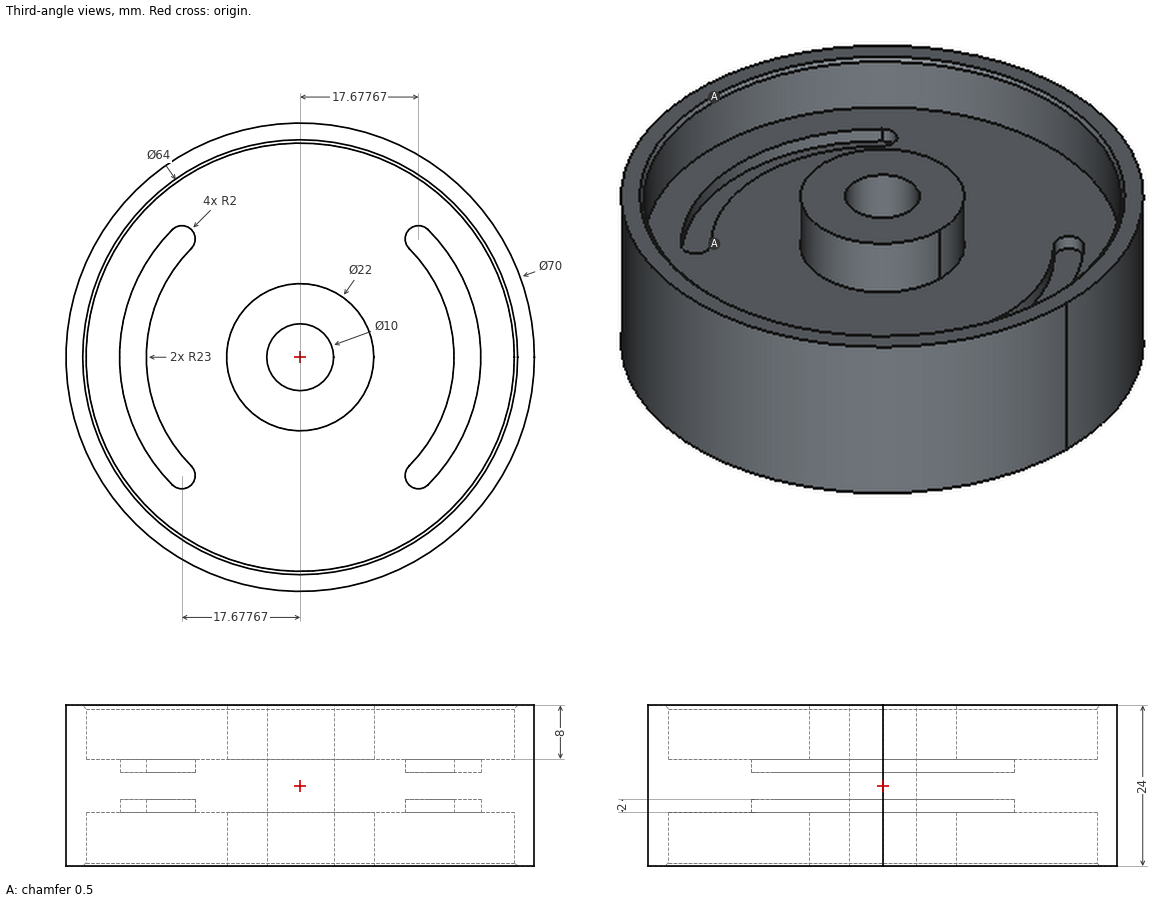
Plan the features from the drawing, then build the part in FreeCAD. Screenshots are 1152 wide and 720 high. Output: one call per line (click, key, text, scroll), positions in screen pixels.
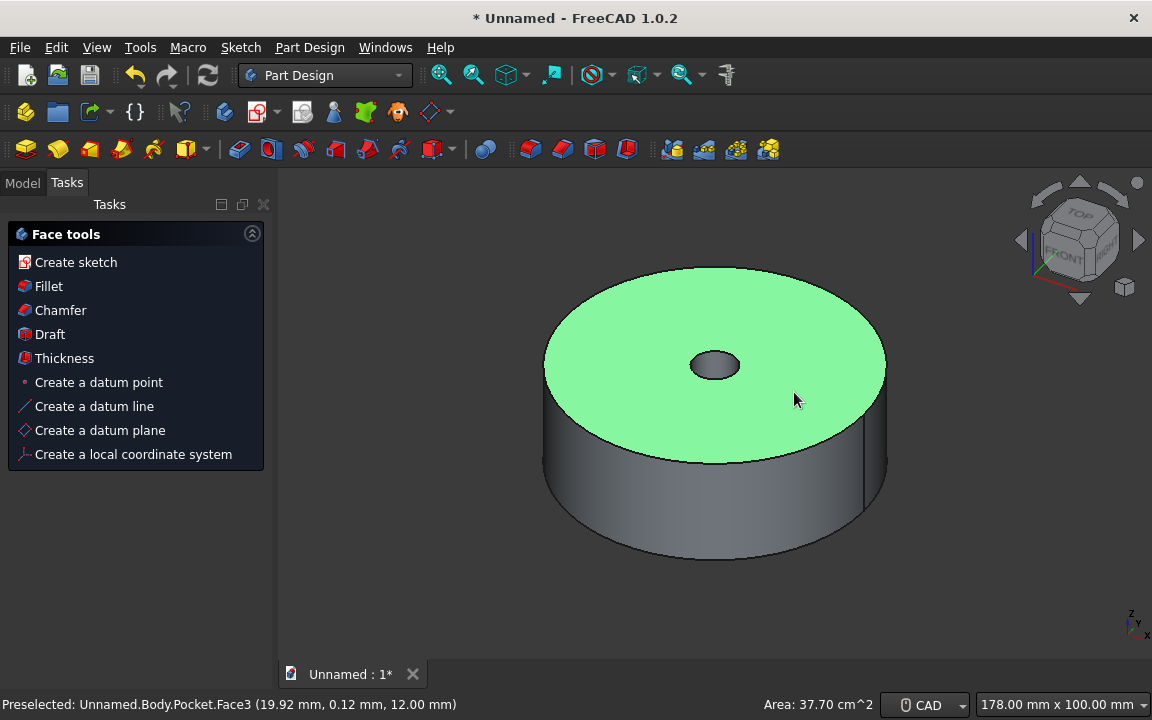
click(258, 112)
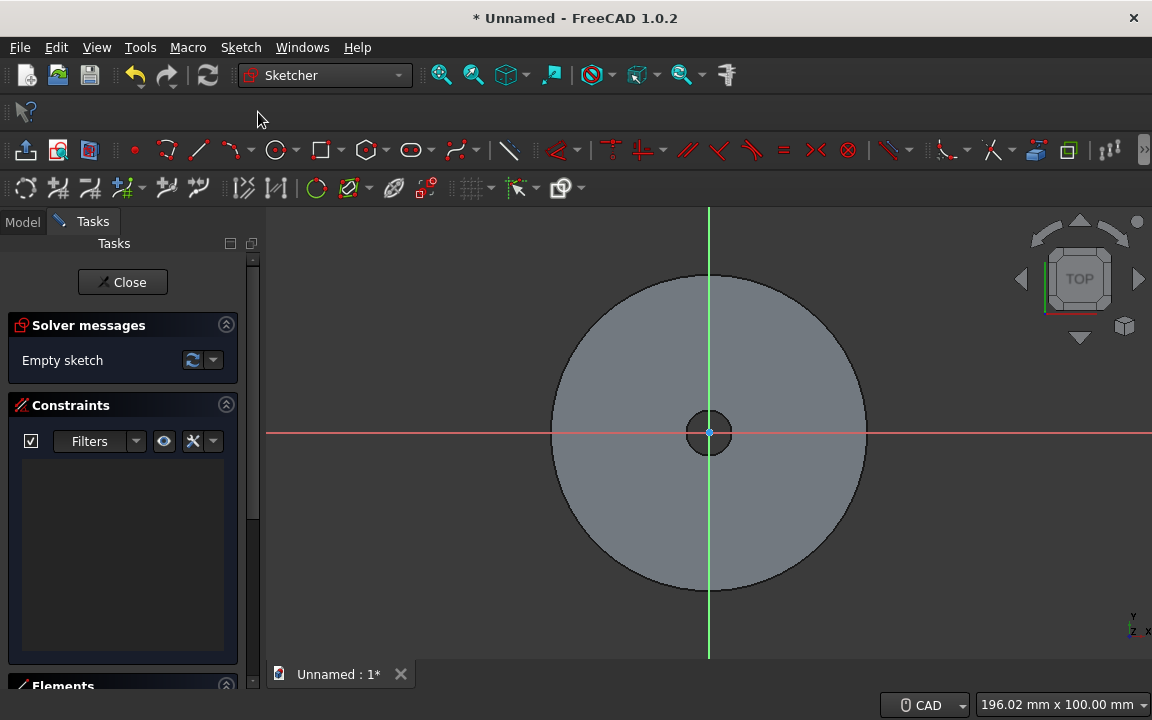
key(g)
key(c)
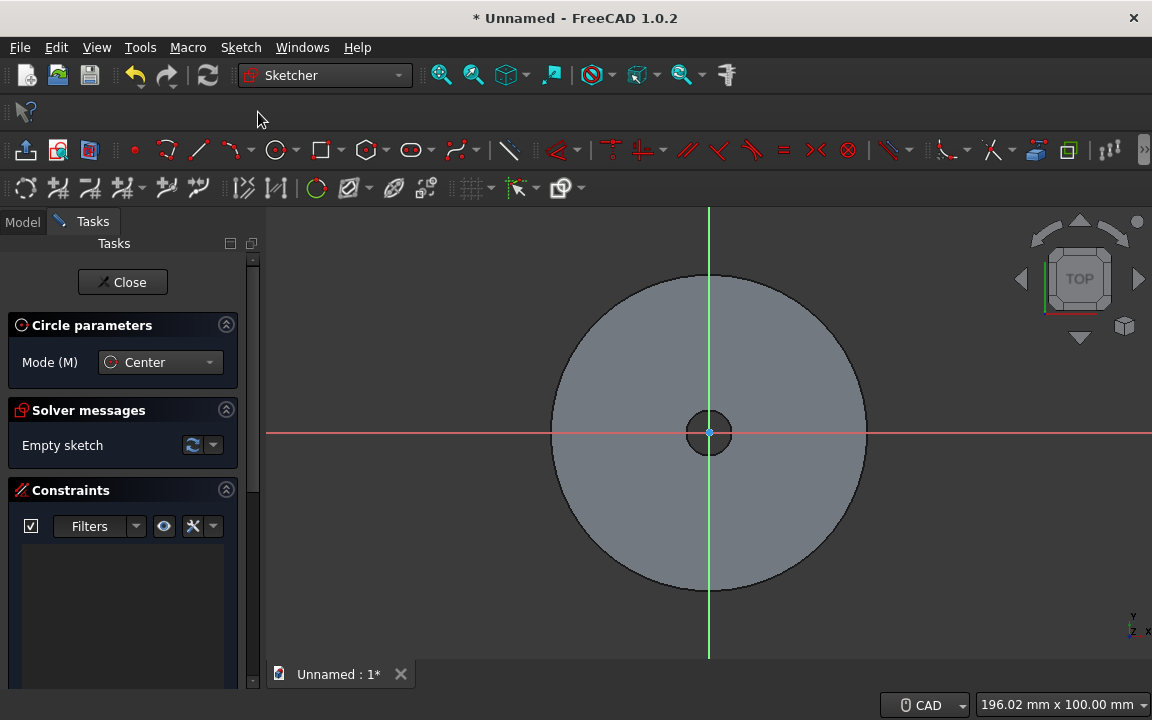
click(709, 433)
move(811, 331)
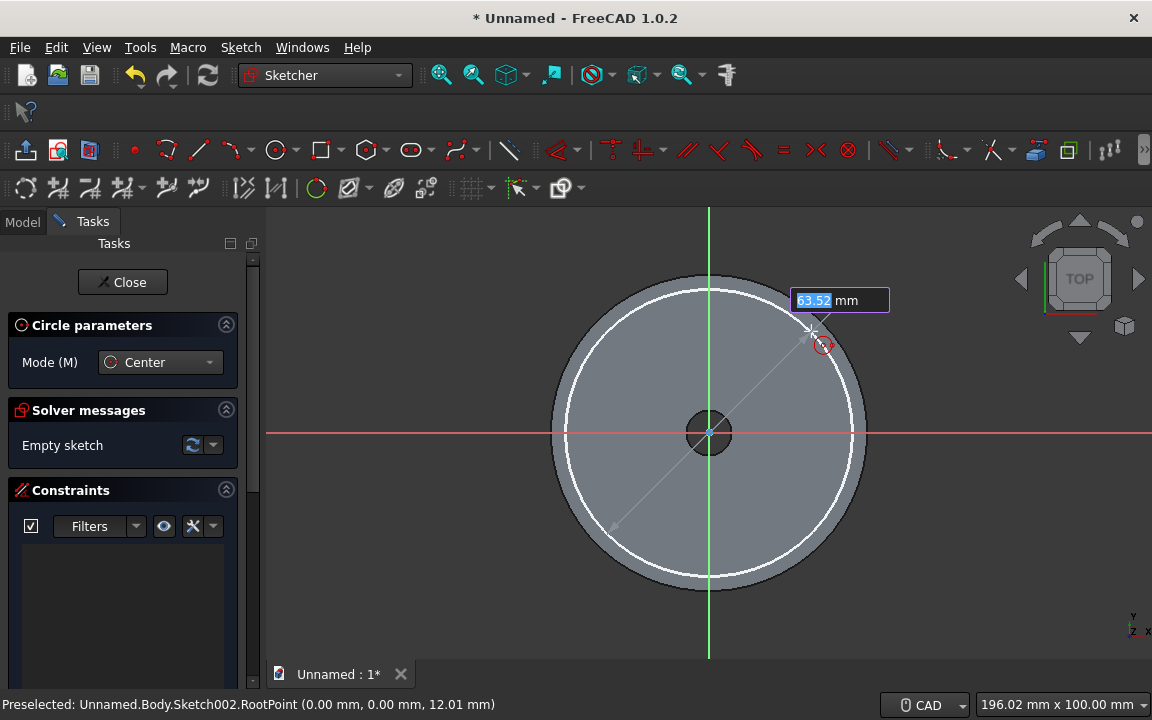
text(64)
key(Return)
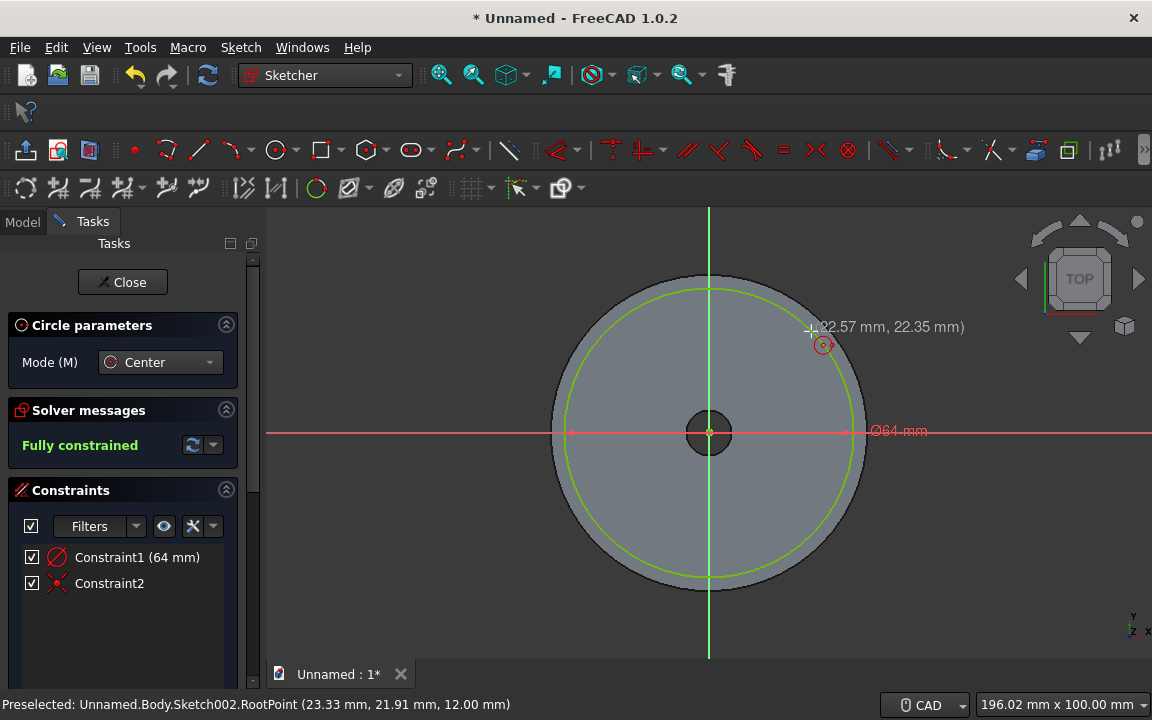
click(709, 433)
move(744, 398)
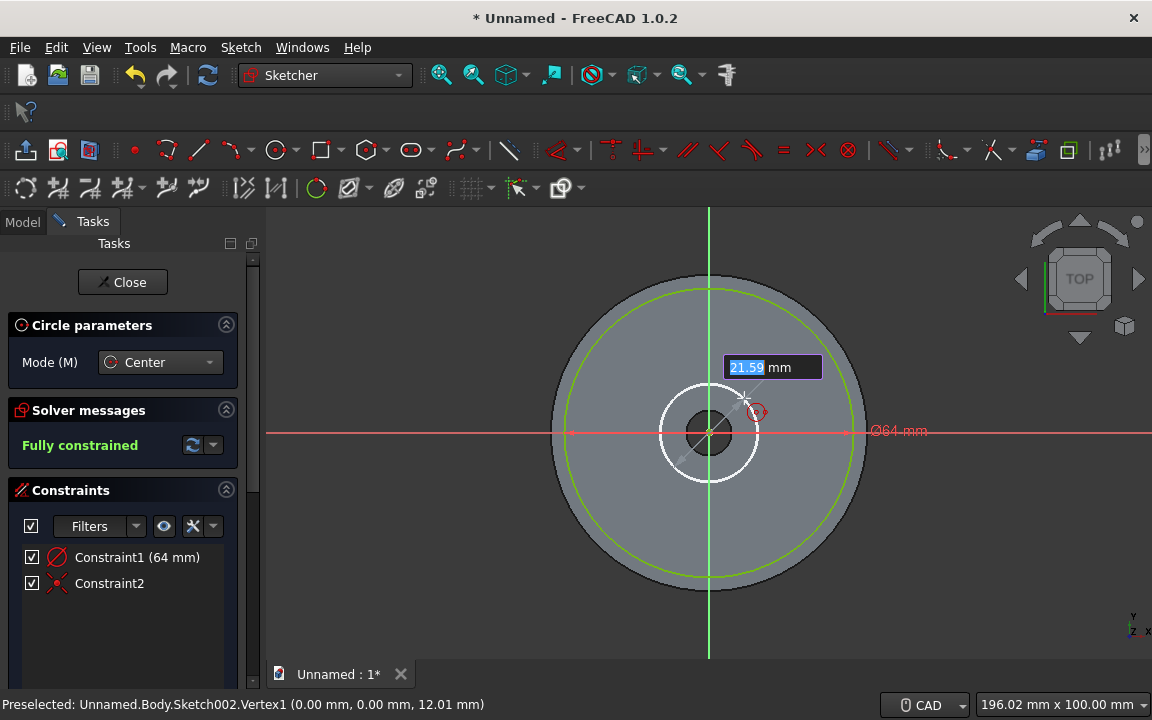
text(22)
key(Return)
key(Escape)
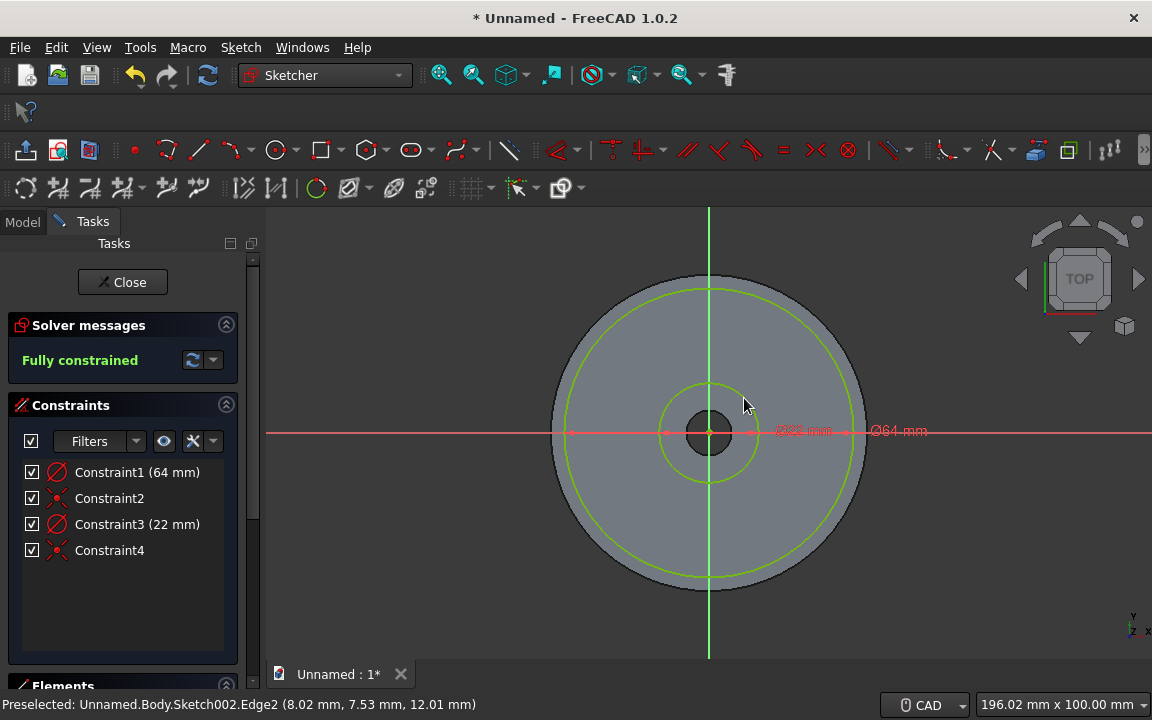
click(123, 282)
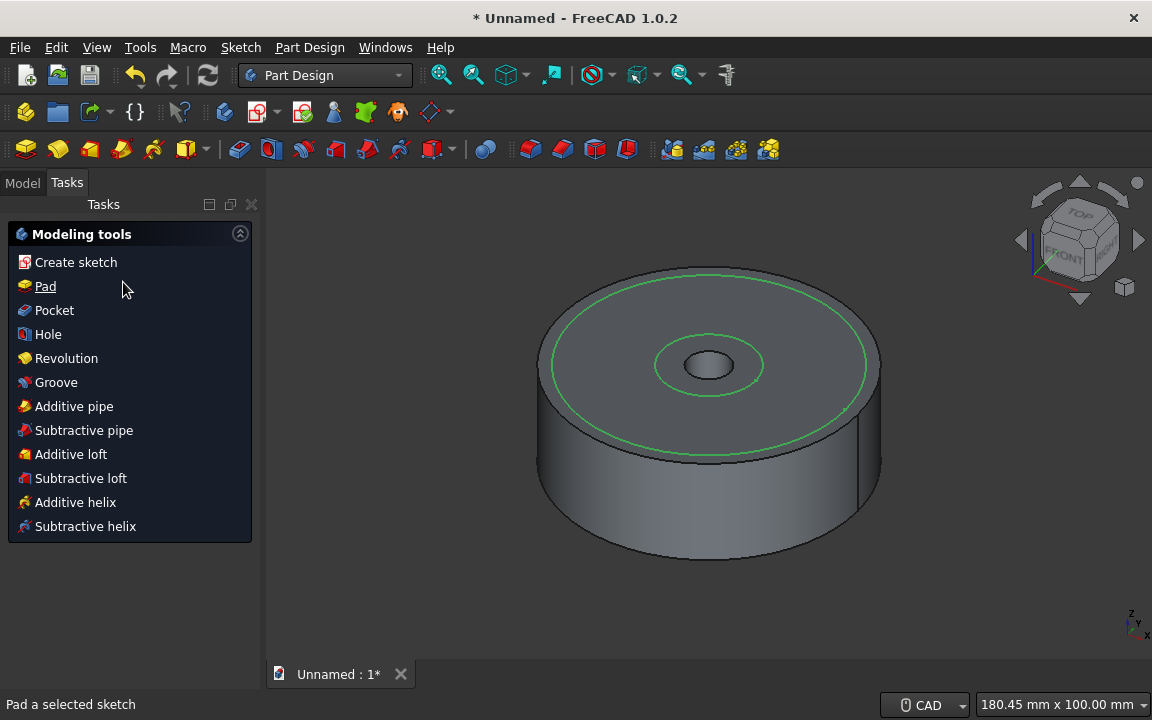
click(240, 150)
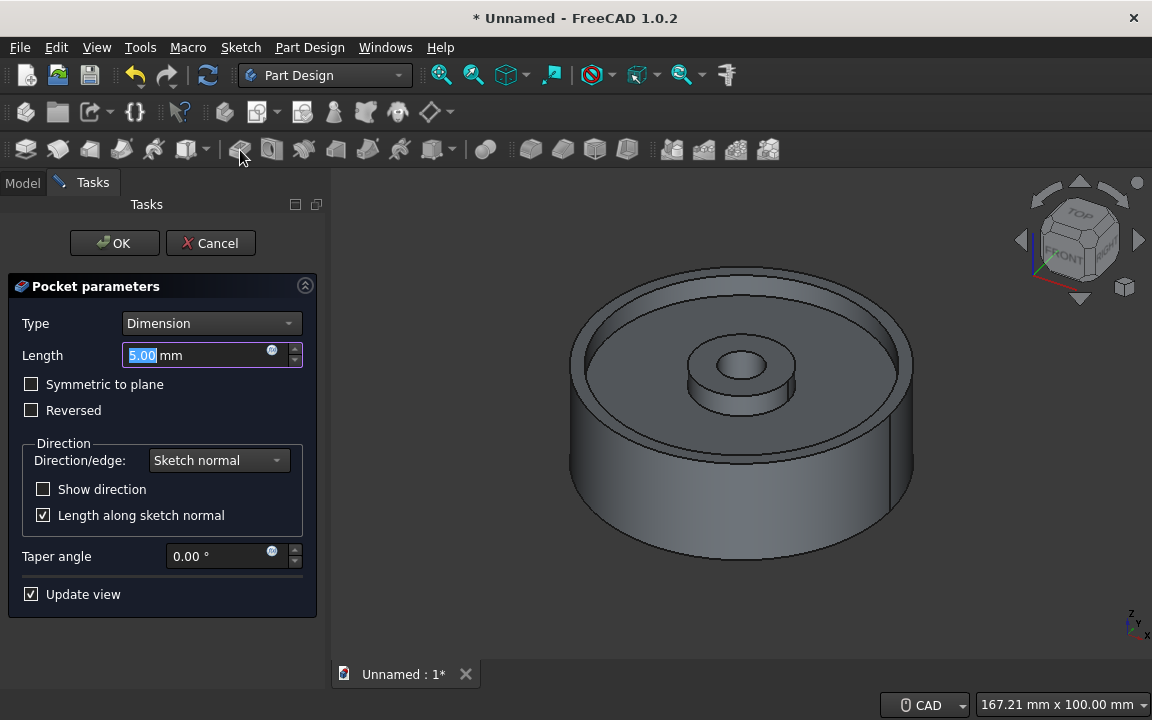
text(8)
key(Tab)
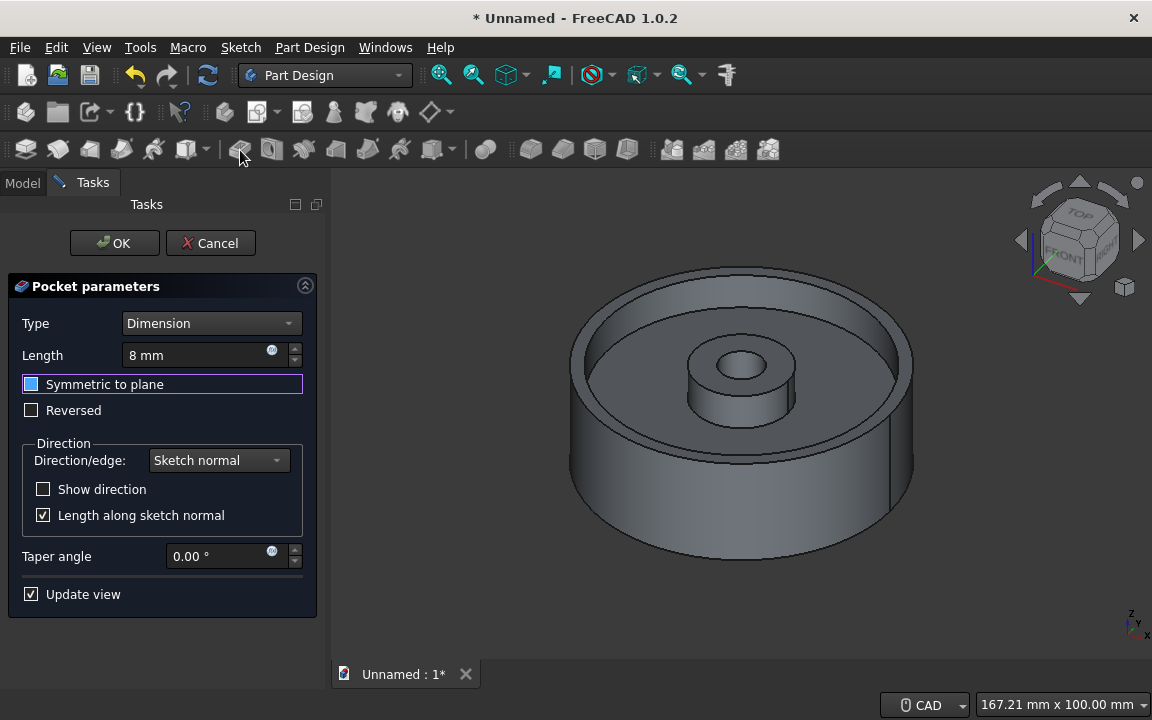
click(115, 243)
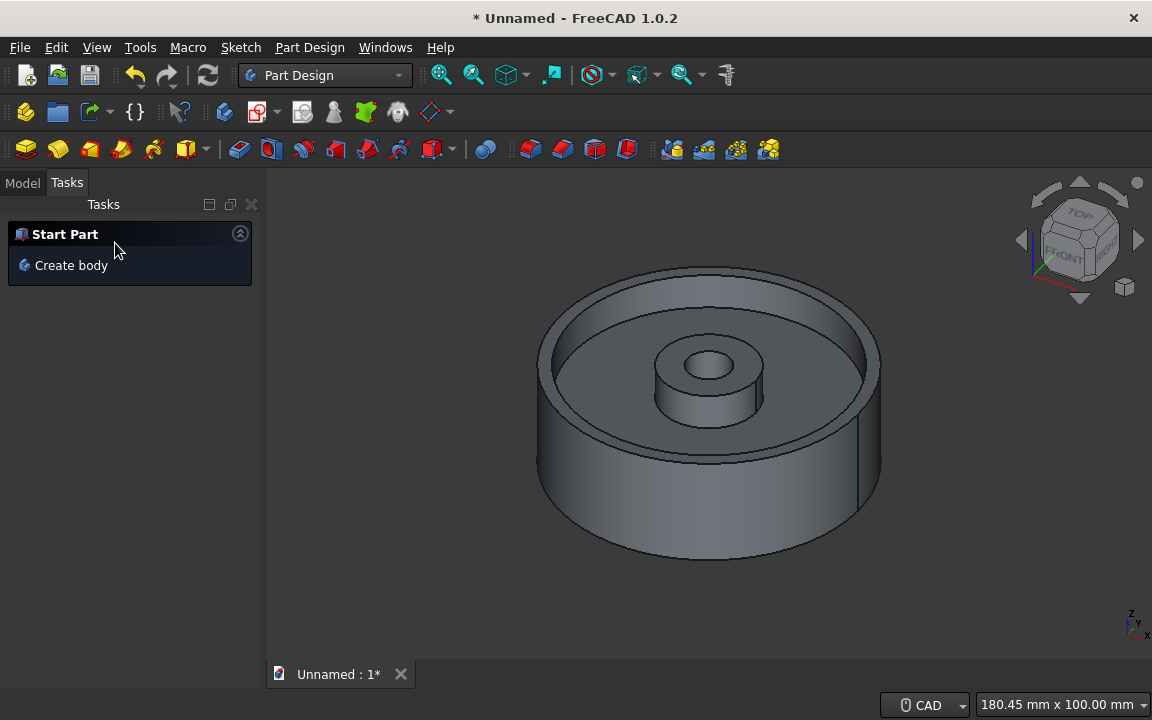
click(23, 182)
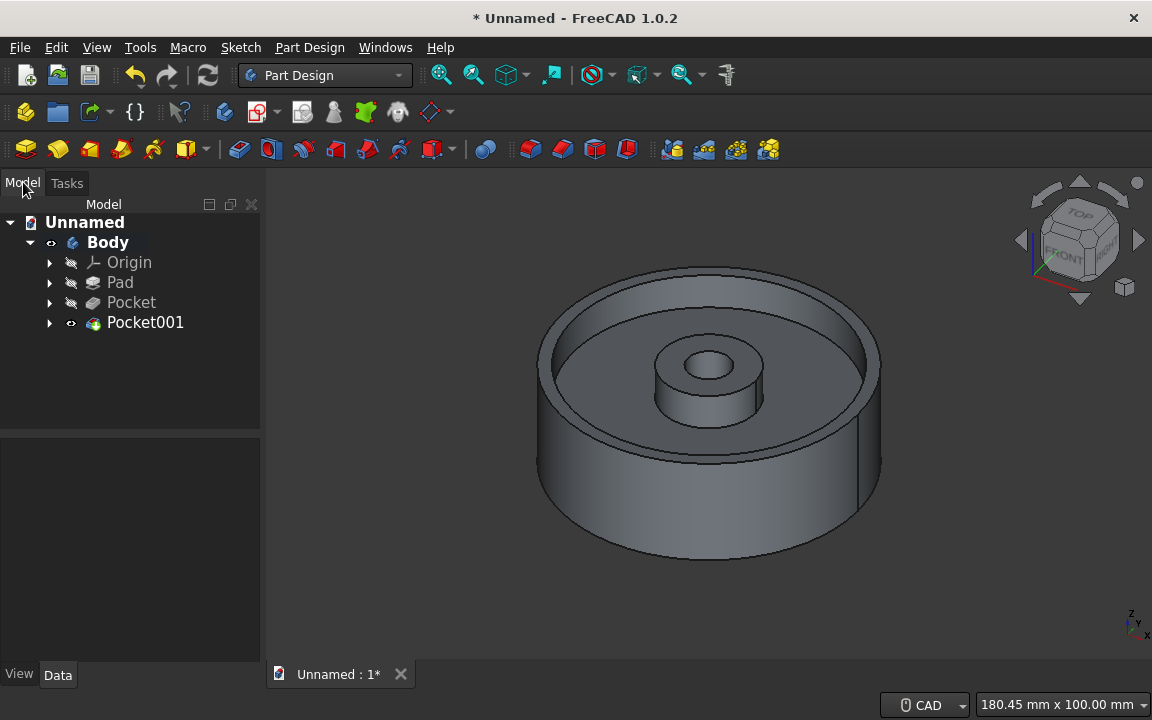
click(116, 323)